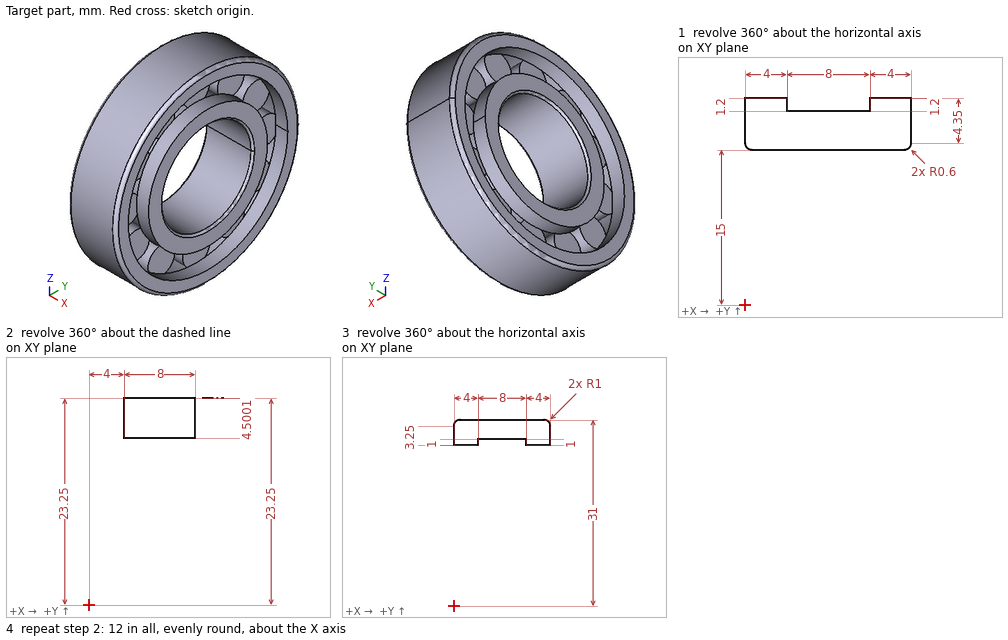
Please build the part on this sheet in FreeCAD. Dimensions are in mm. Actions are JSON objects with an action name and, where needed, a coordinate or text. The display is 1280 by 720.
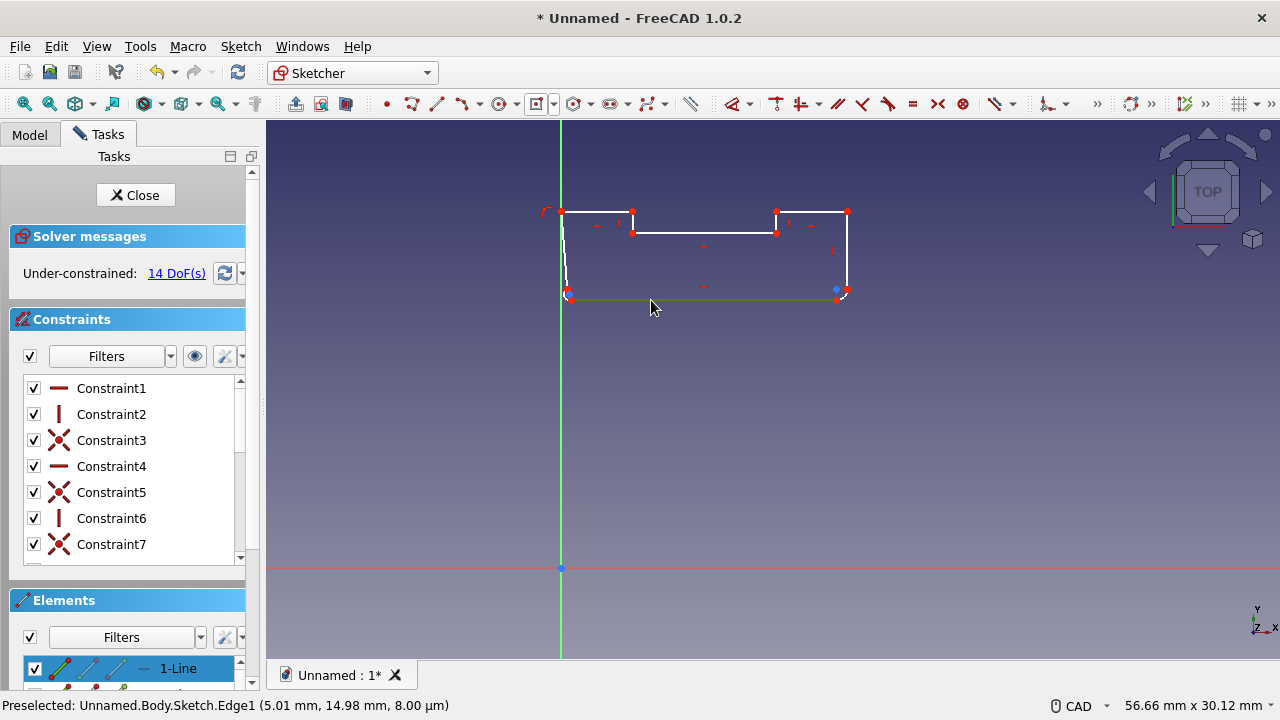
{"action": "scroll", "coordinate": [844, 297], "scroll_direction": "up", "scroll_amount": 3}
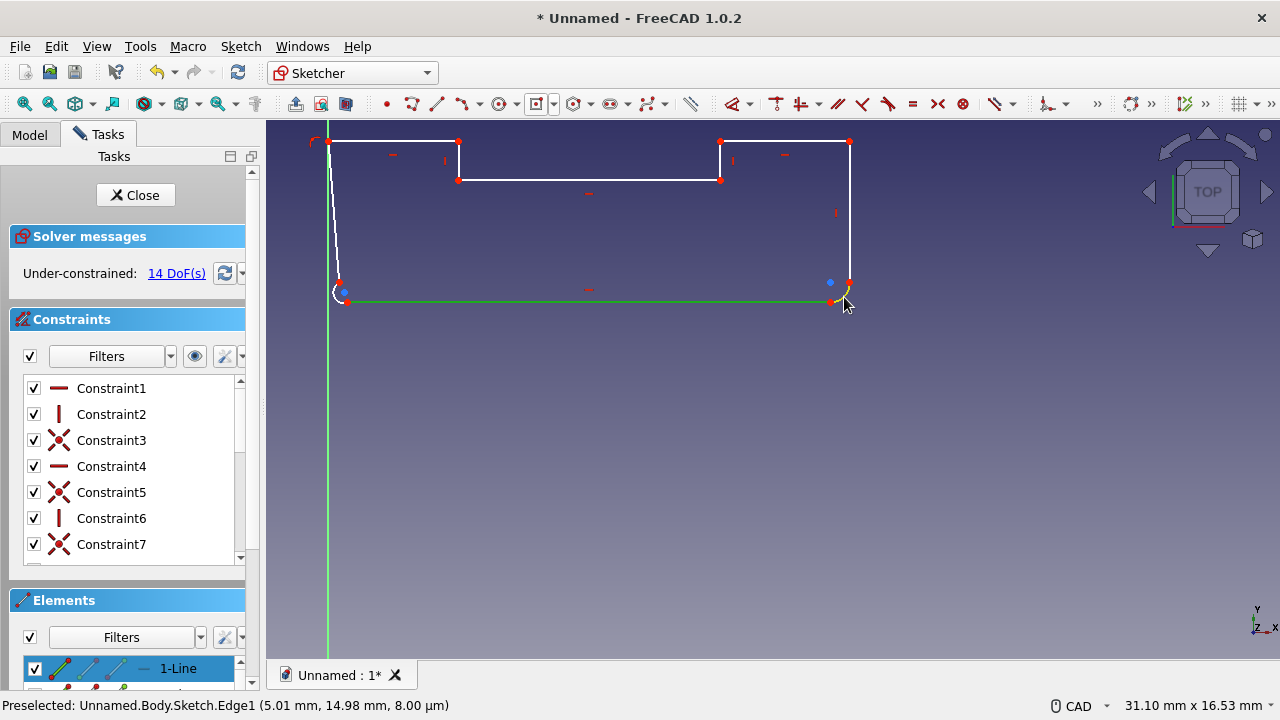
{"action": "left_click", "coordinate": [844, 297]}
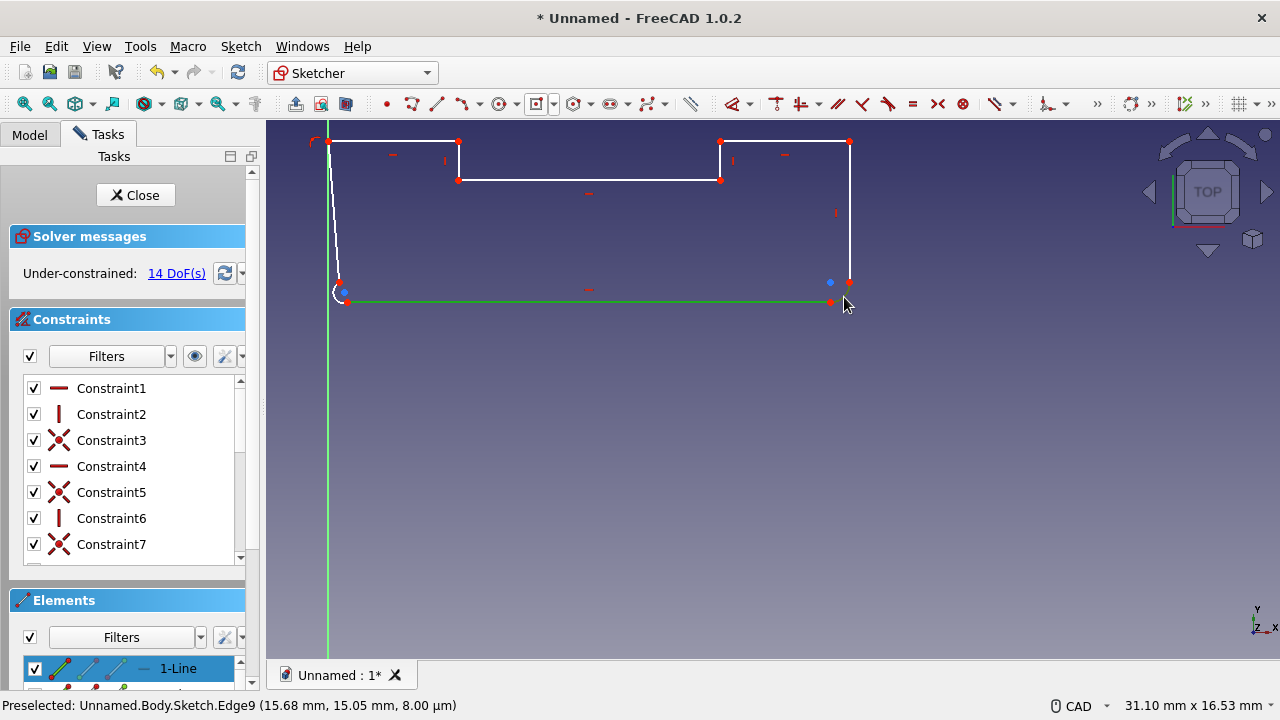
{"action": "key", "text": "t"}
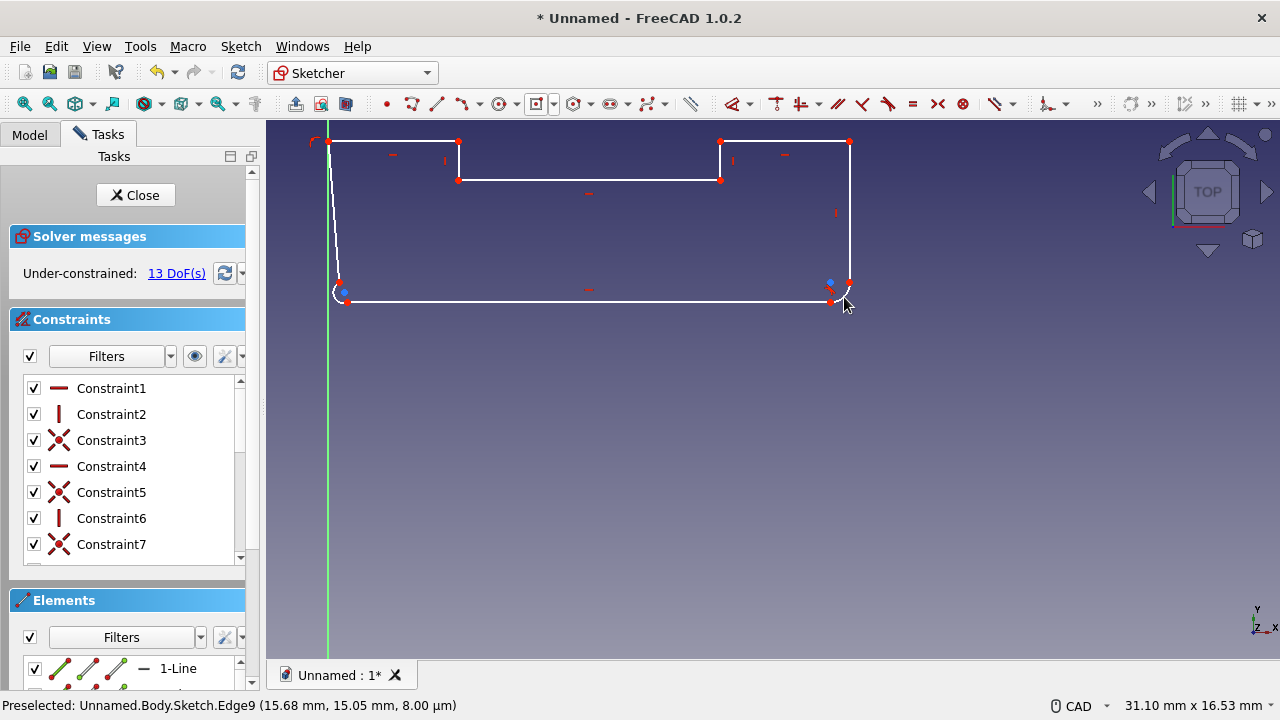
{"action": "left_click", "coordinate": [493, 302]}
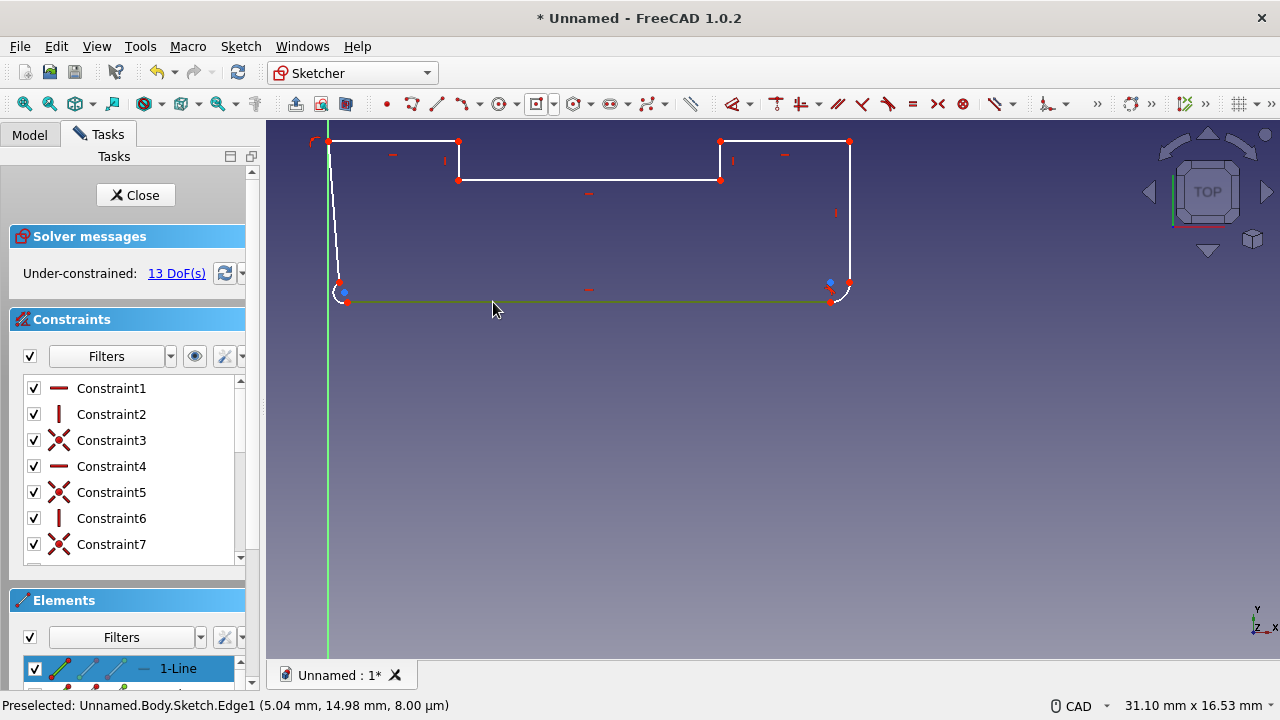
{"action": "scroll", "coordinate": [338, 302], "scroll_direction": "up", "scroll_amount": 2}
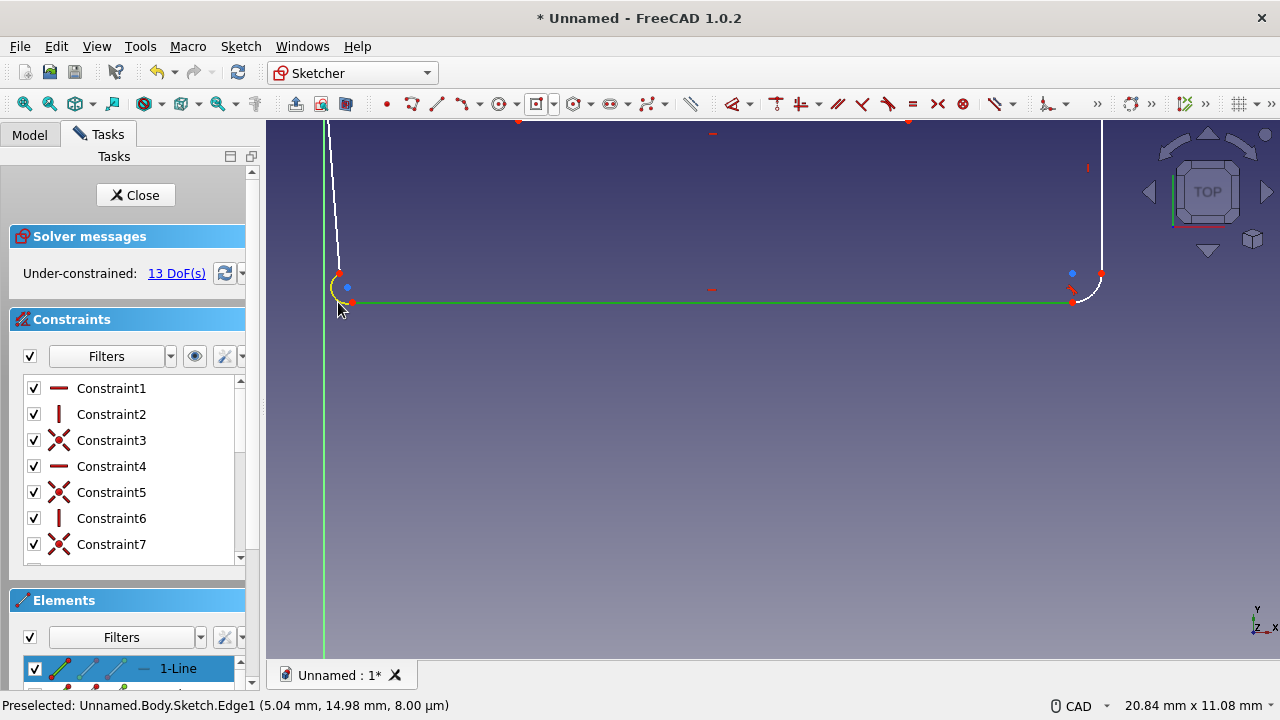
{"action": "left_click", "coordinate": [339, 301]}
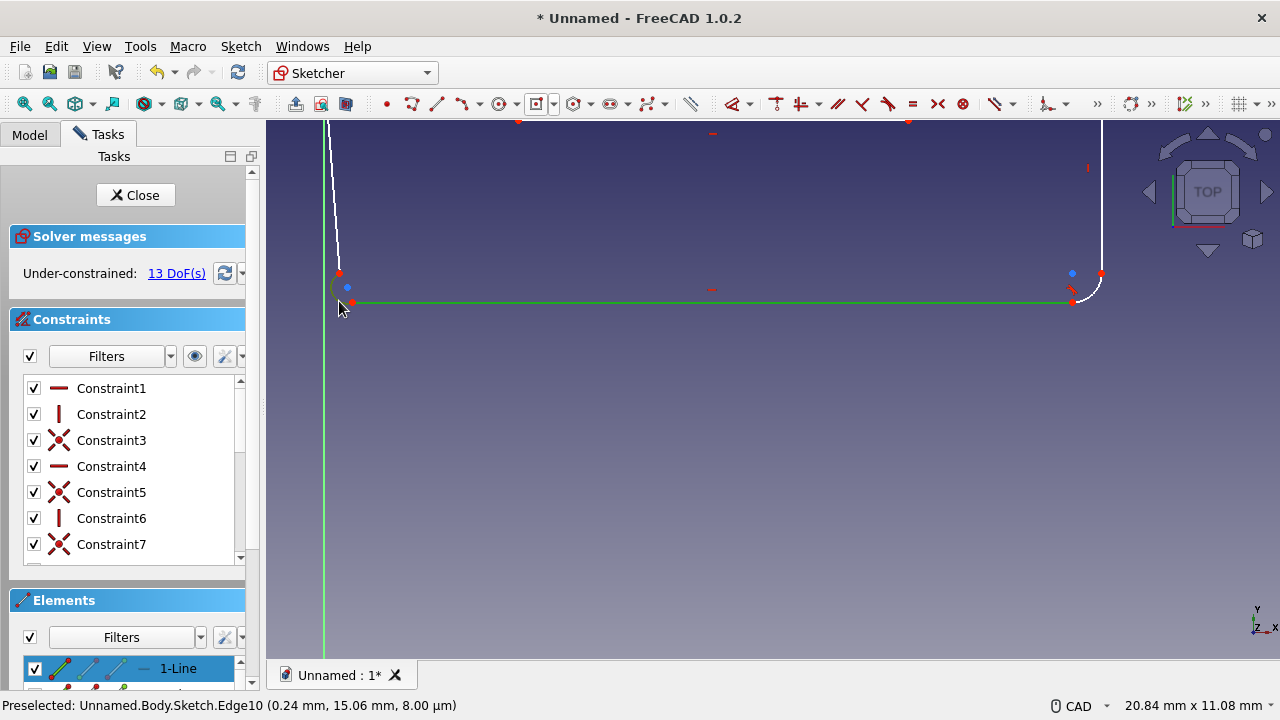
{"action": "left_click", "coordinate": [888, 104]}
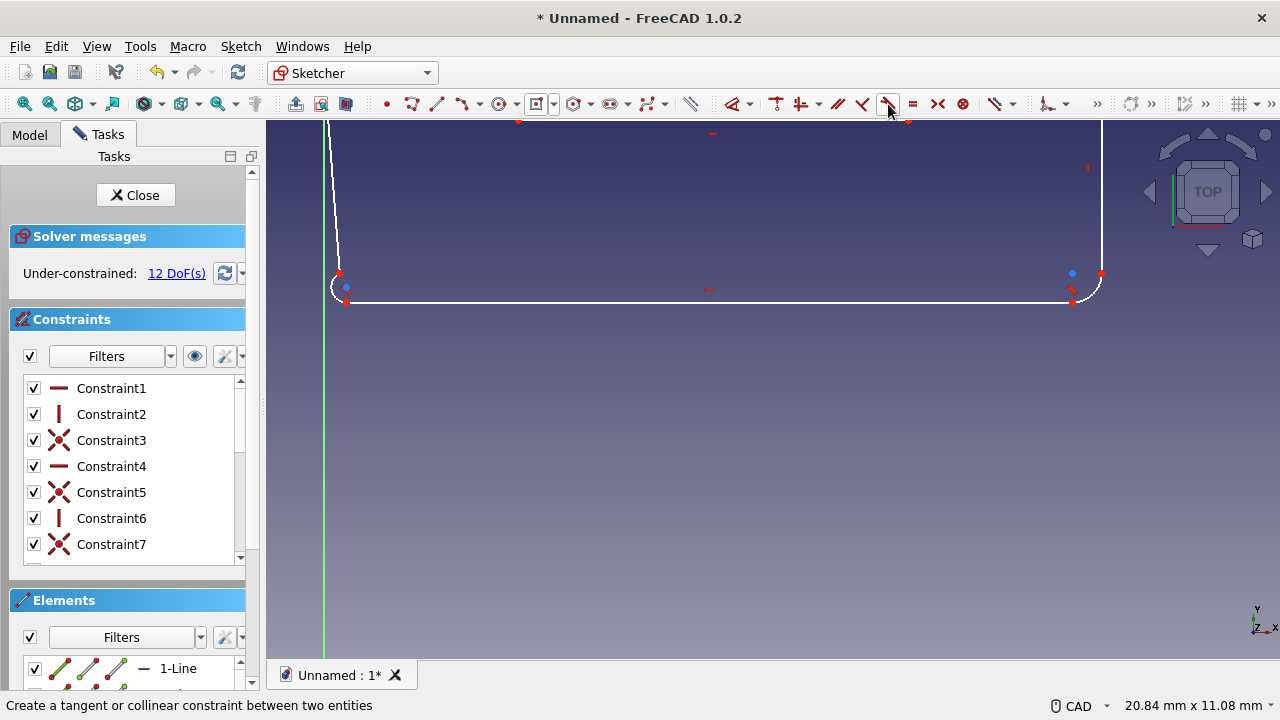
{"action": "left_click", "coordinate": [1102, 210]}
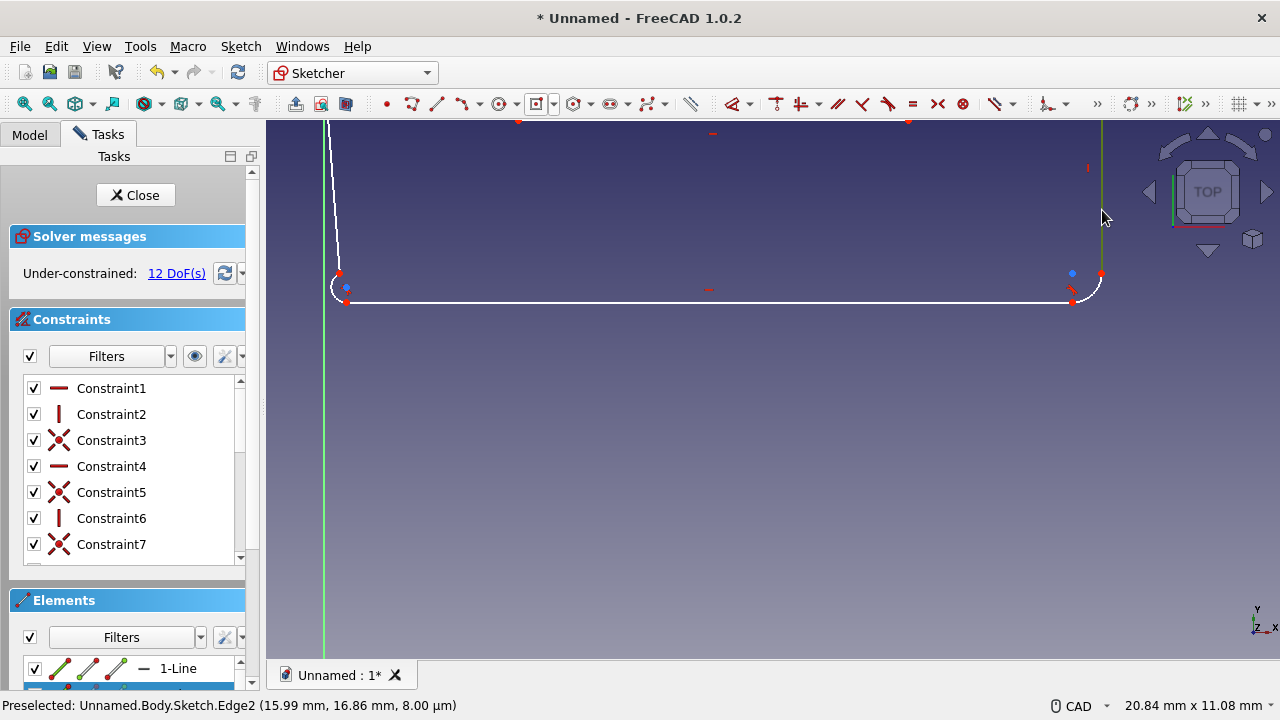
{"action": "left_click", "coordinate": [1086, 299]}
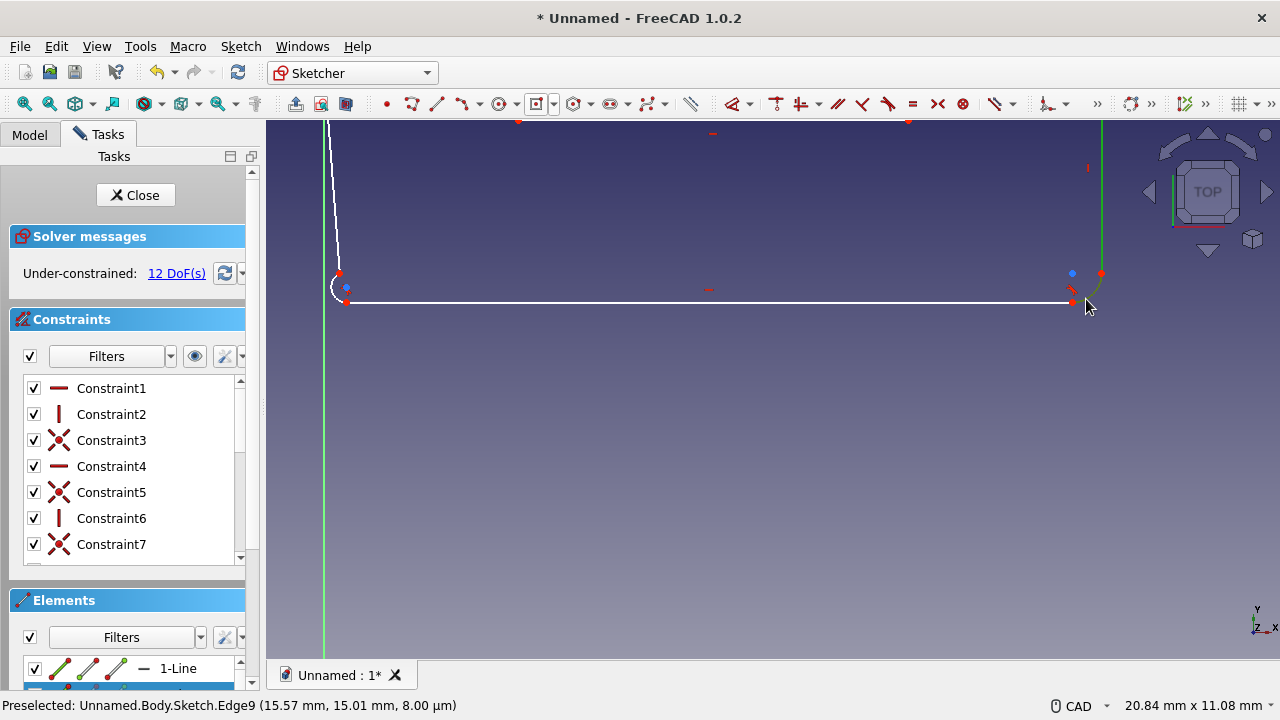
{"action": "left_click", "coordinate": [888, 104]}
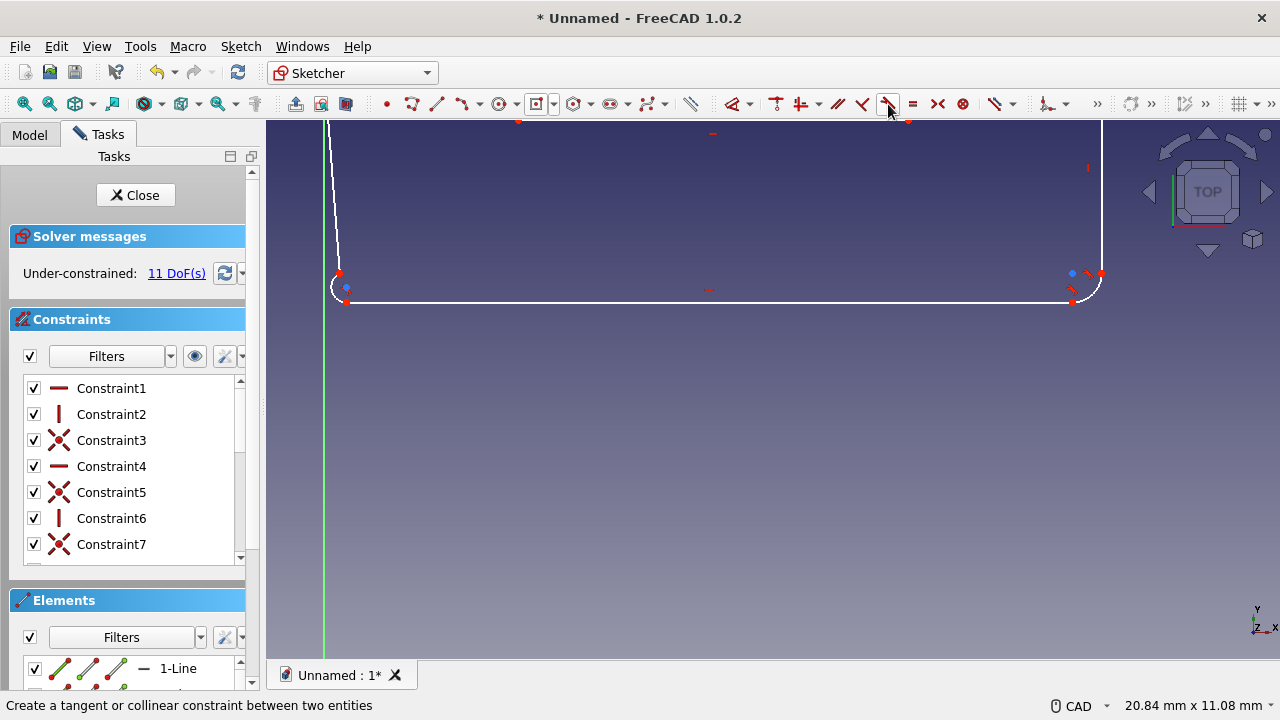
{"action": "scroll", "coordinate": [335, 210], "scroll_direction": "up", "scroll_amount": 2}